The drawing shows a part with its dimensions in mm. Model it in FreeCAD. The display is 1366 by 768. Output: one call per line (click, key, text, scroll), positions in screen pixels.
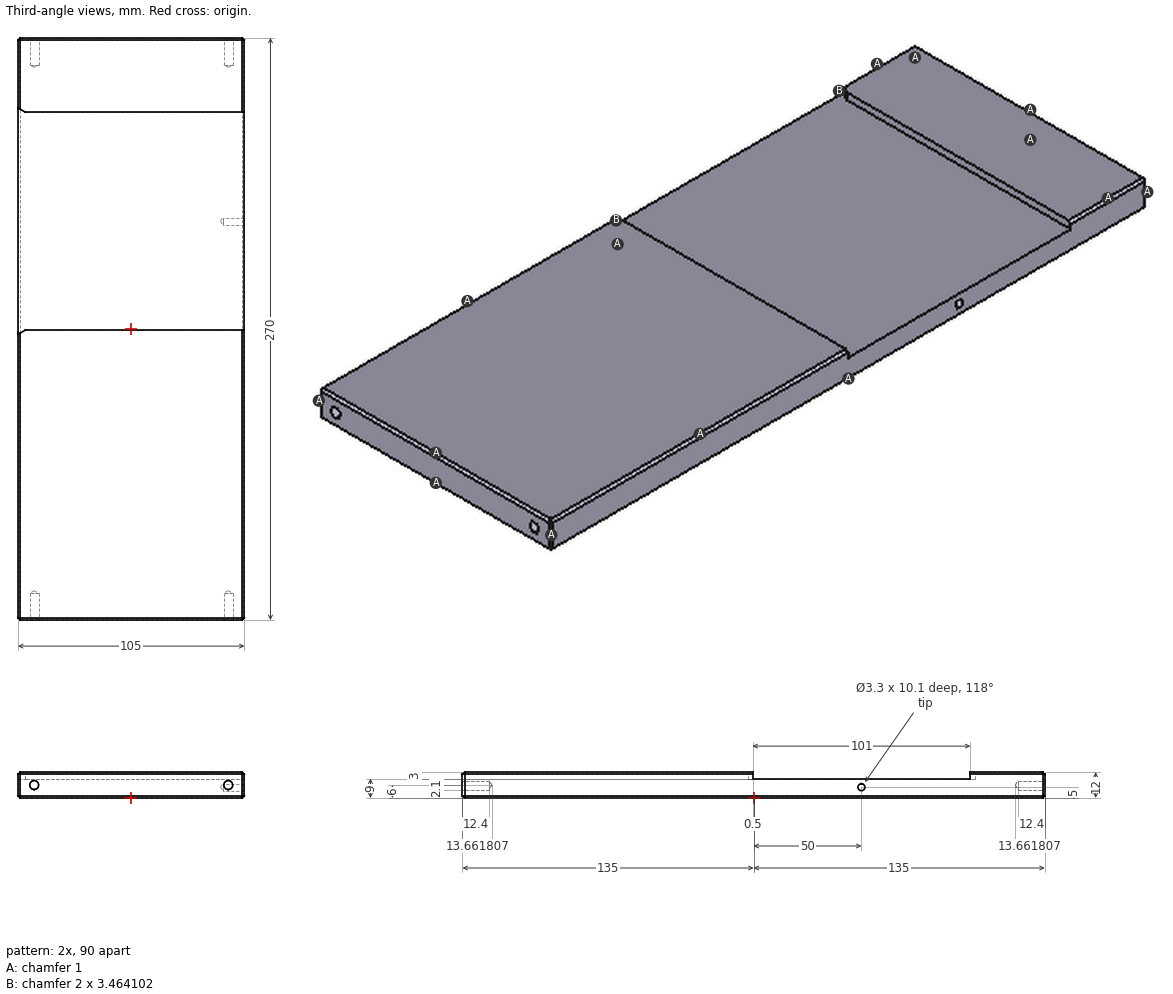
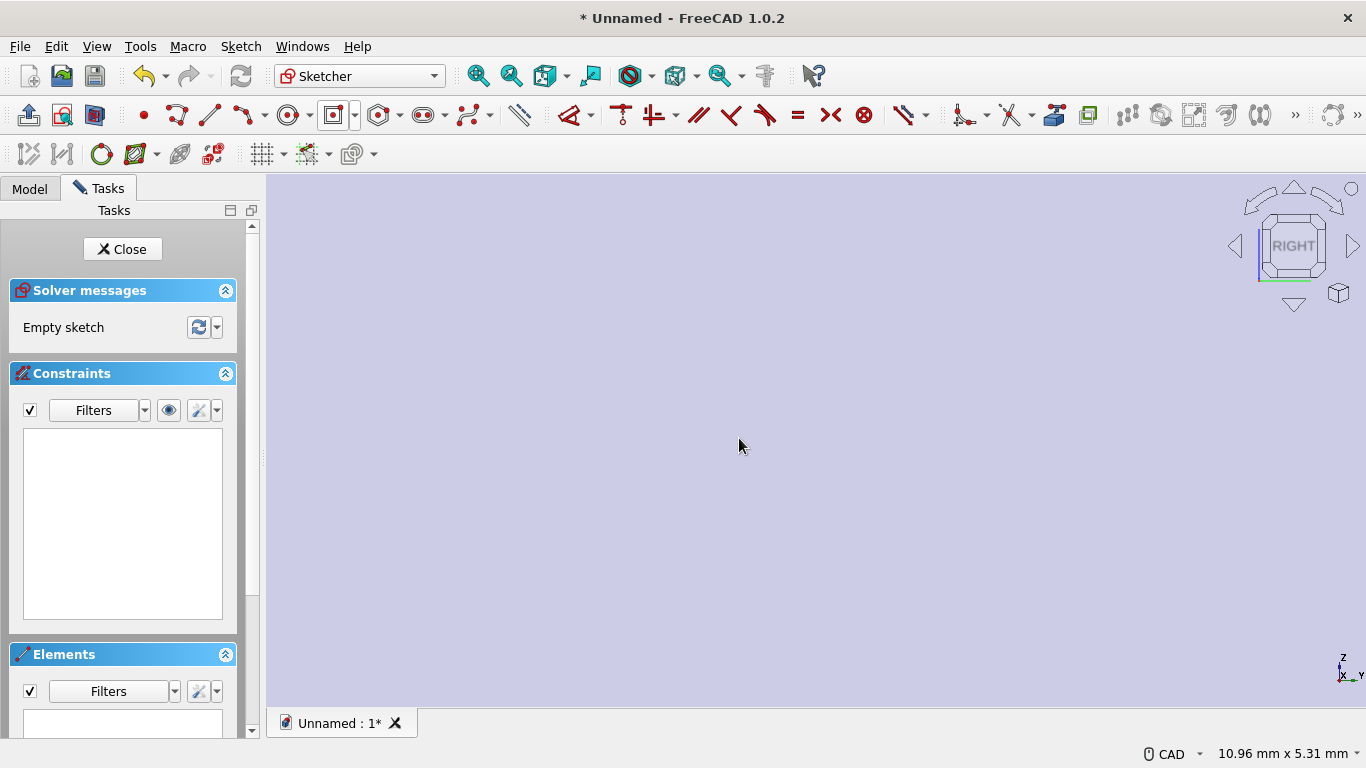
click(288, 116)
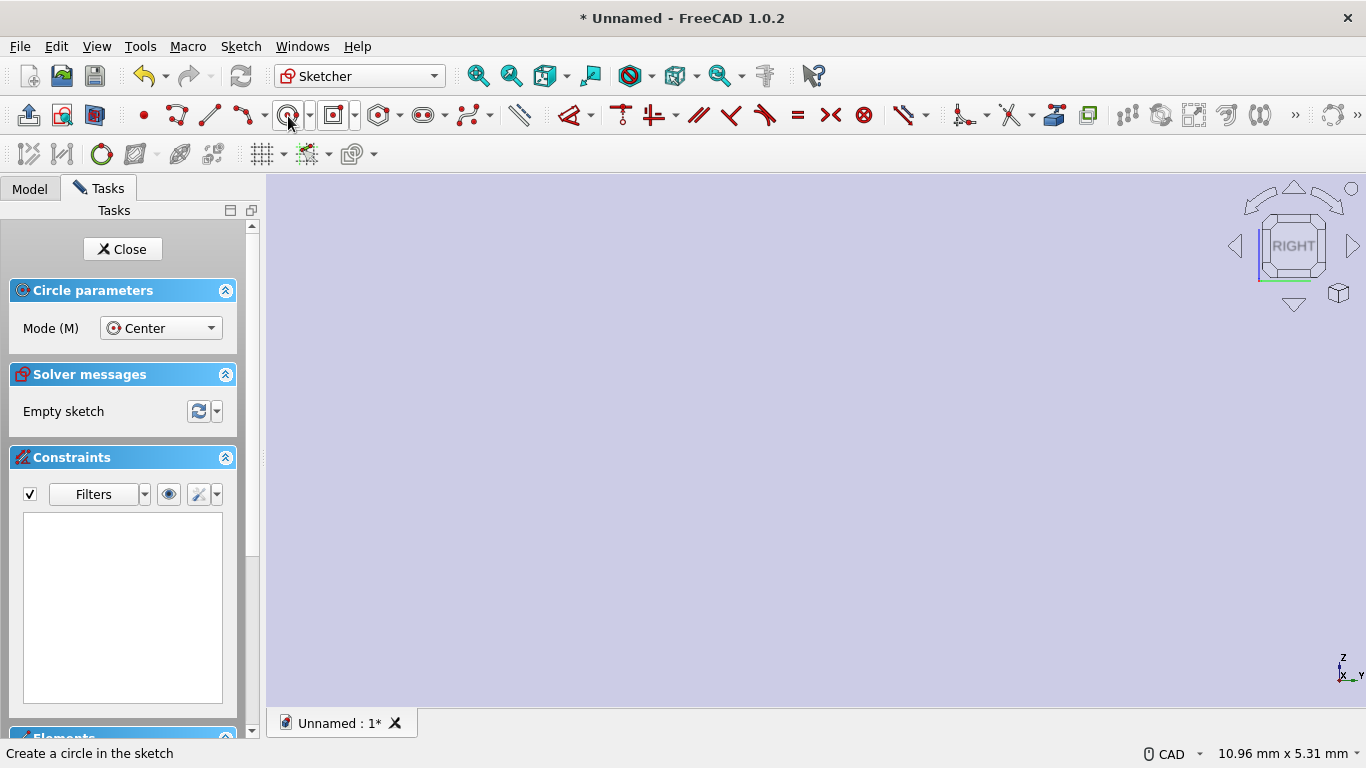
click(747, 440)
move(864, 323)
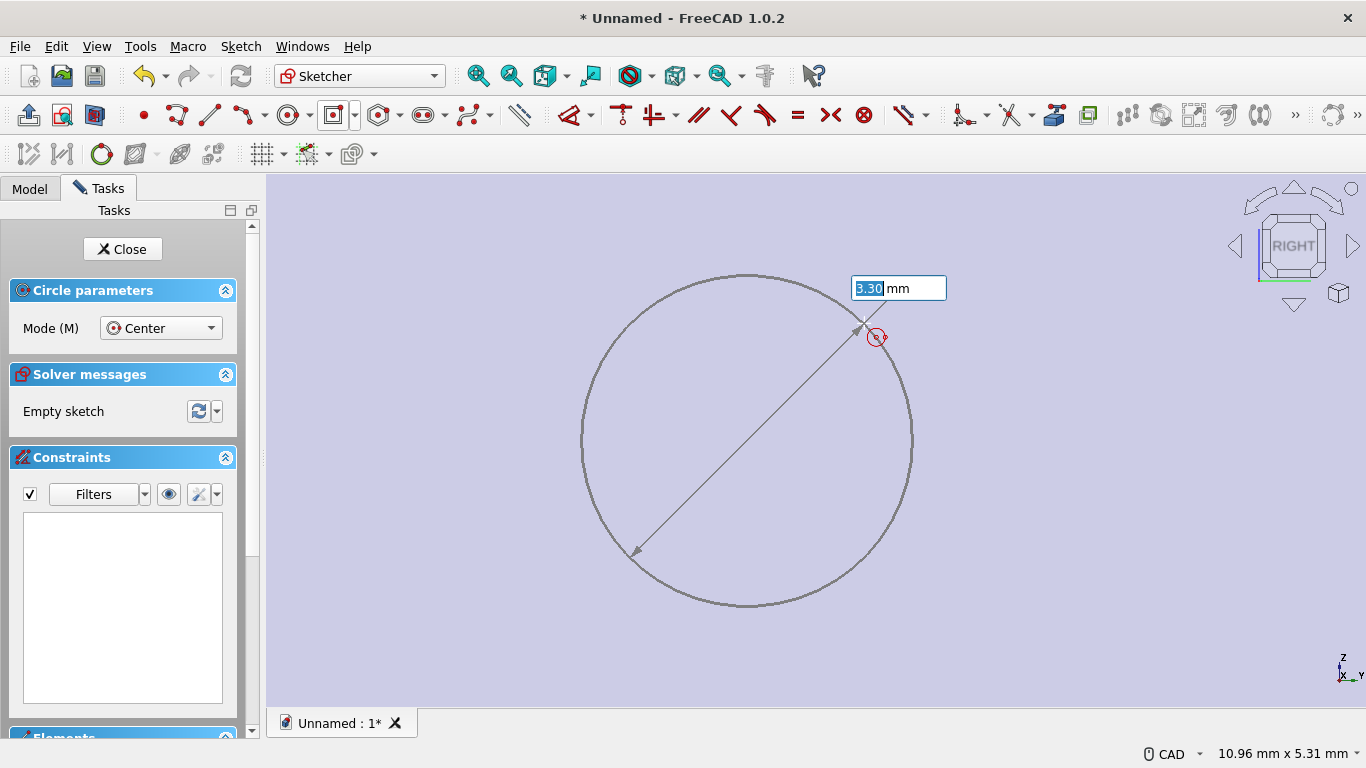
text(3.3)
key(Return)
key(Escape)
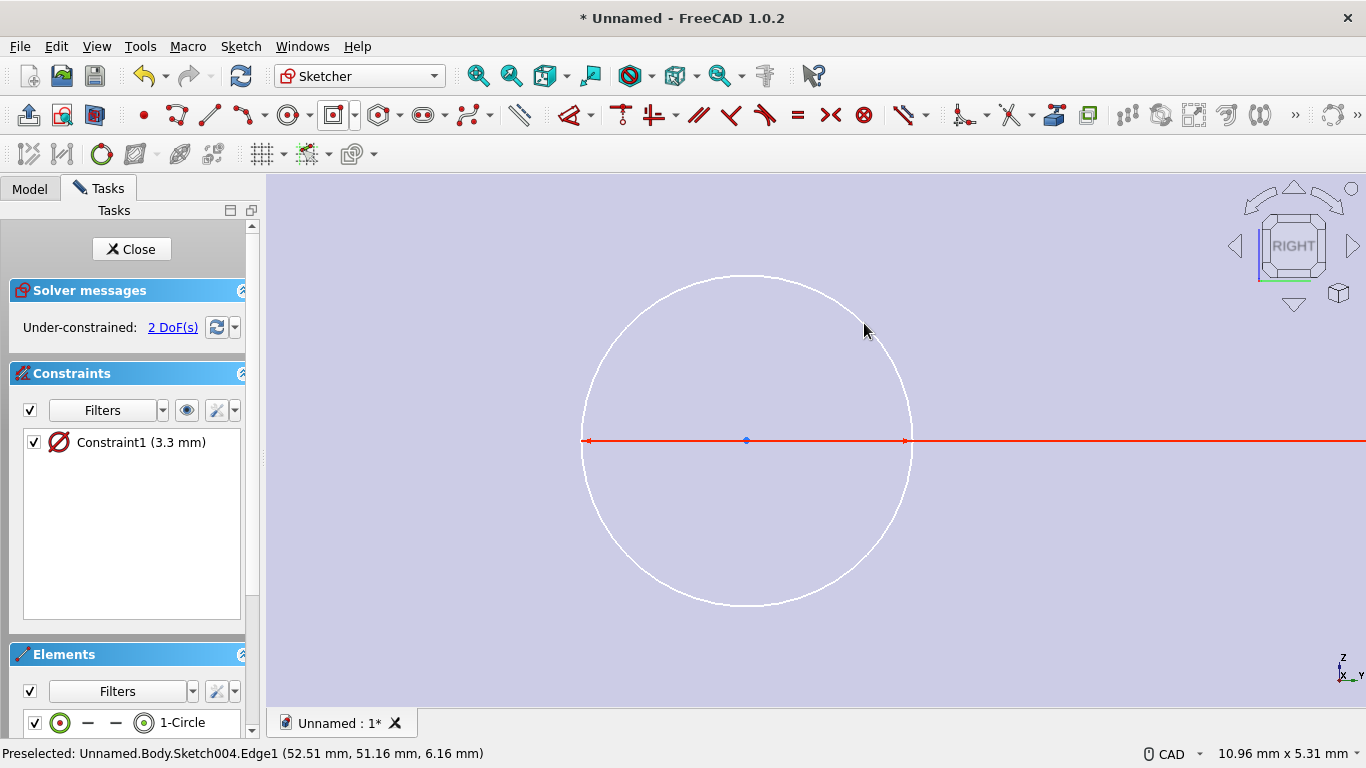
click(568, 116)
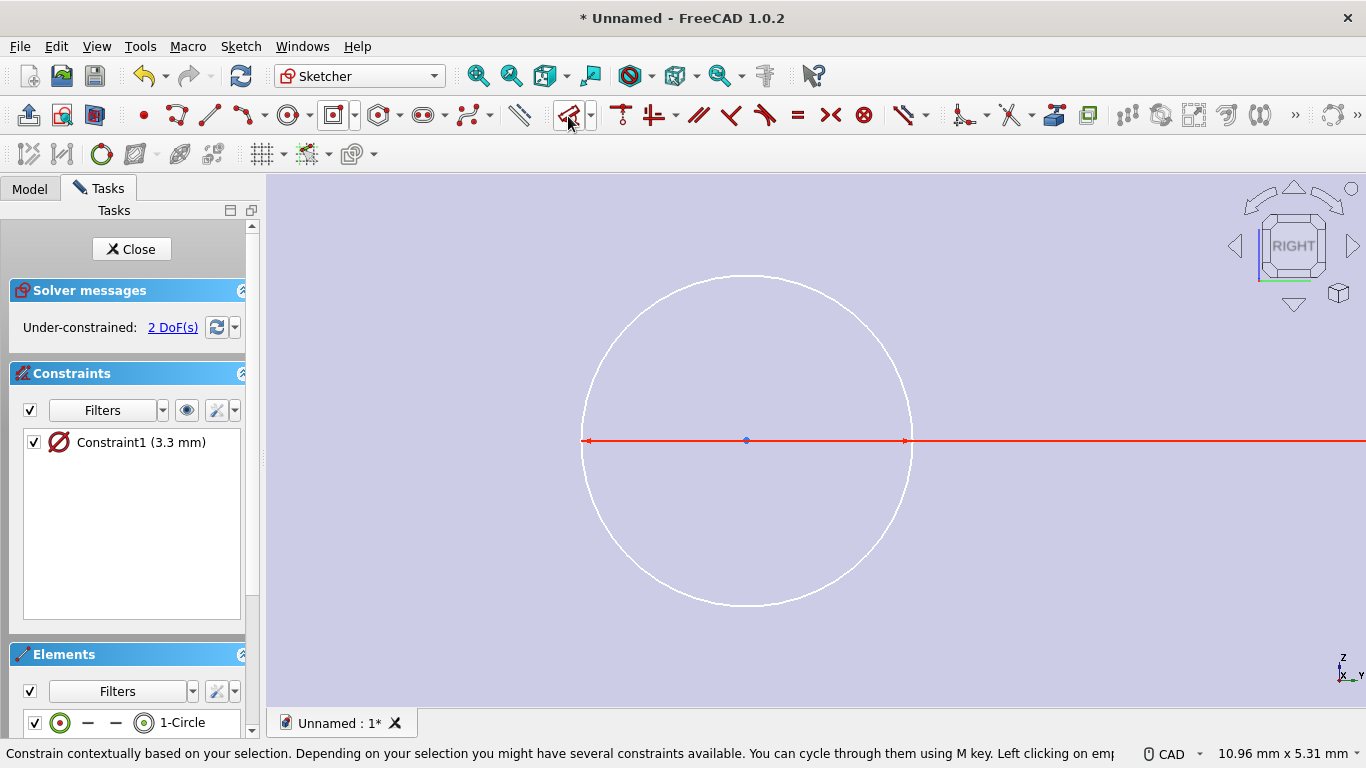
click(747, 441)
click(781, 560)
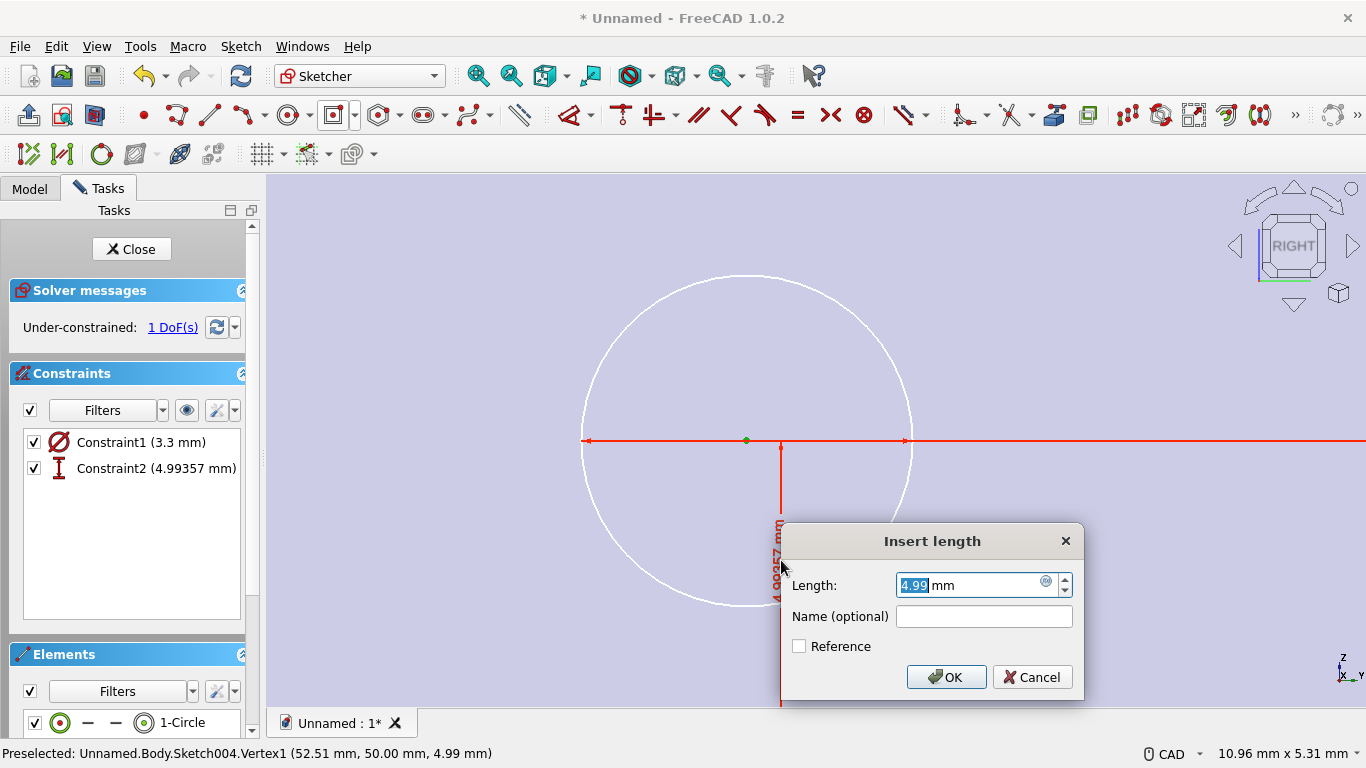
text(5)
key(Return)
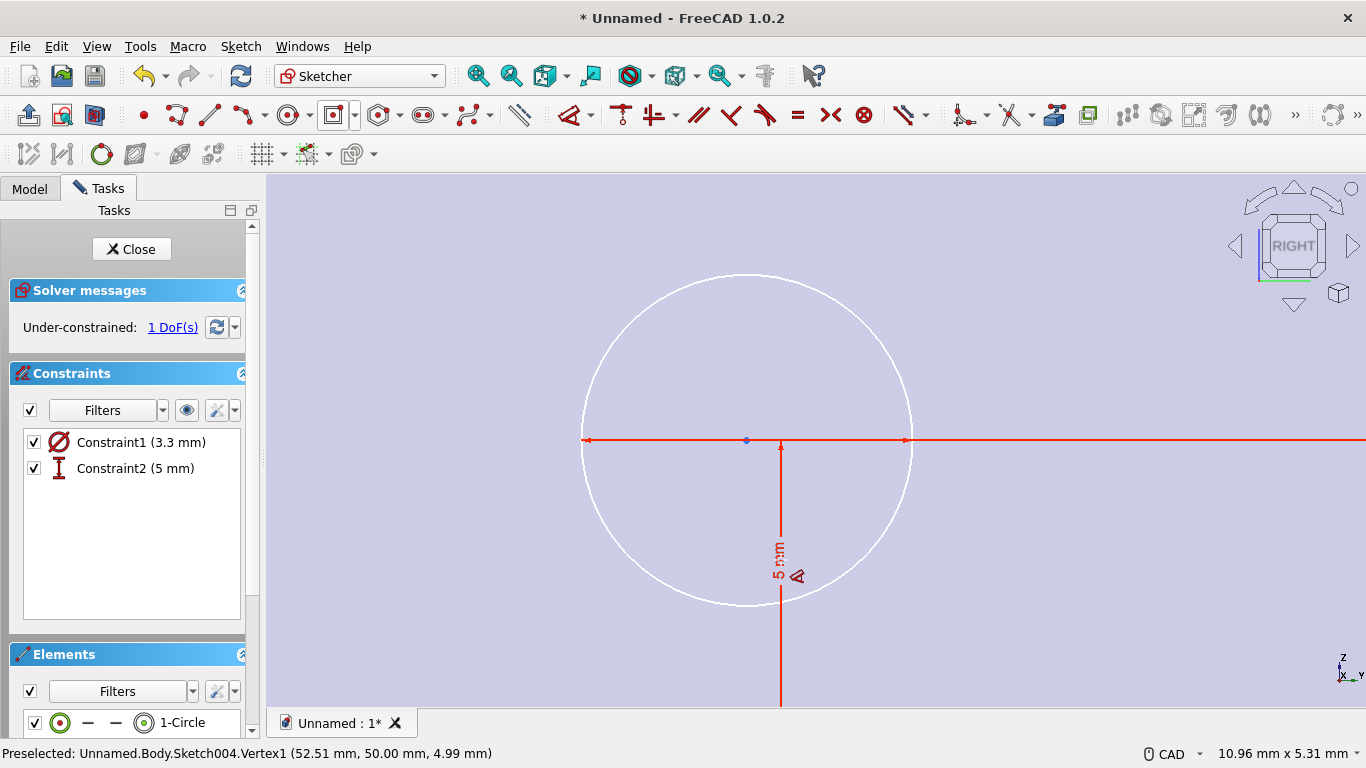
click(747, 440)
click(520, 406)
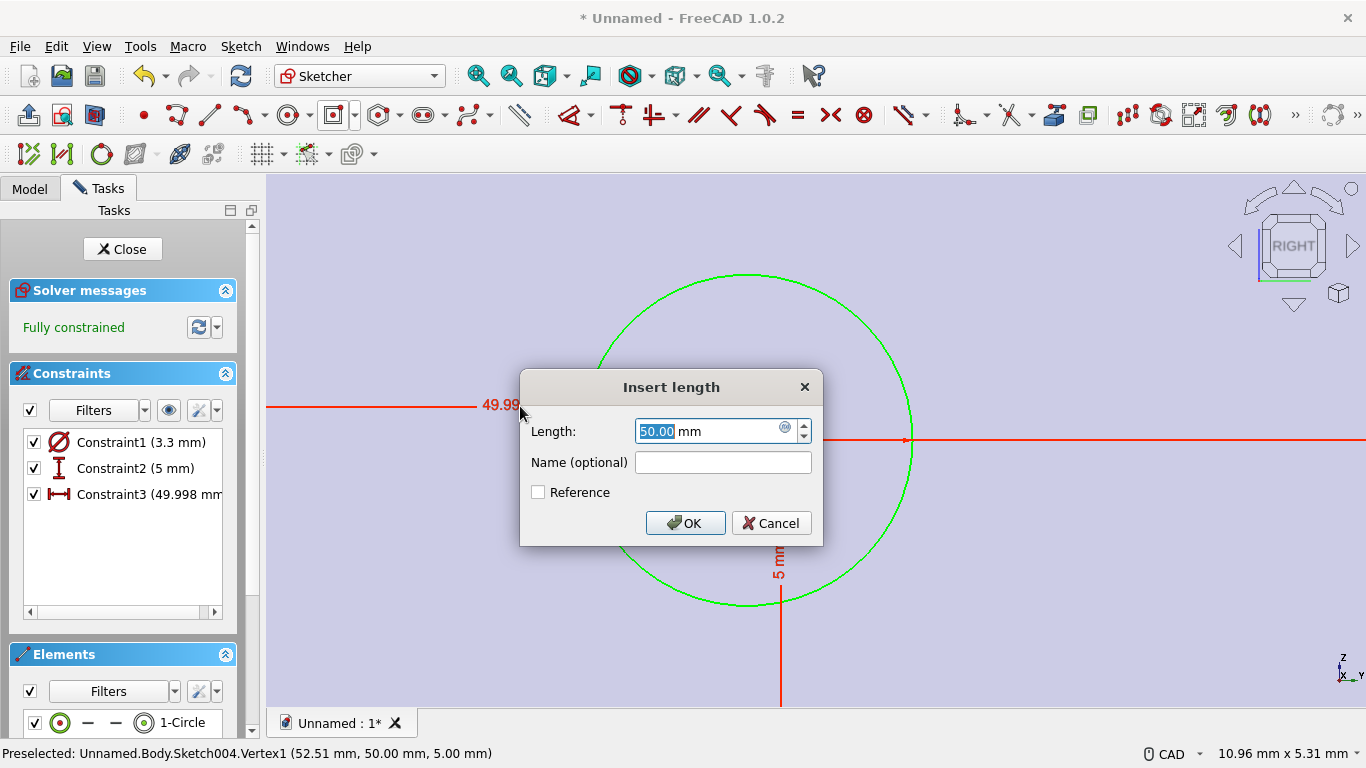
text(50)
key(Return)
key(Escape)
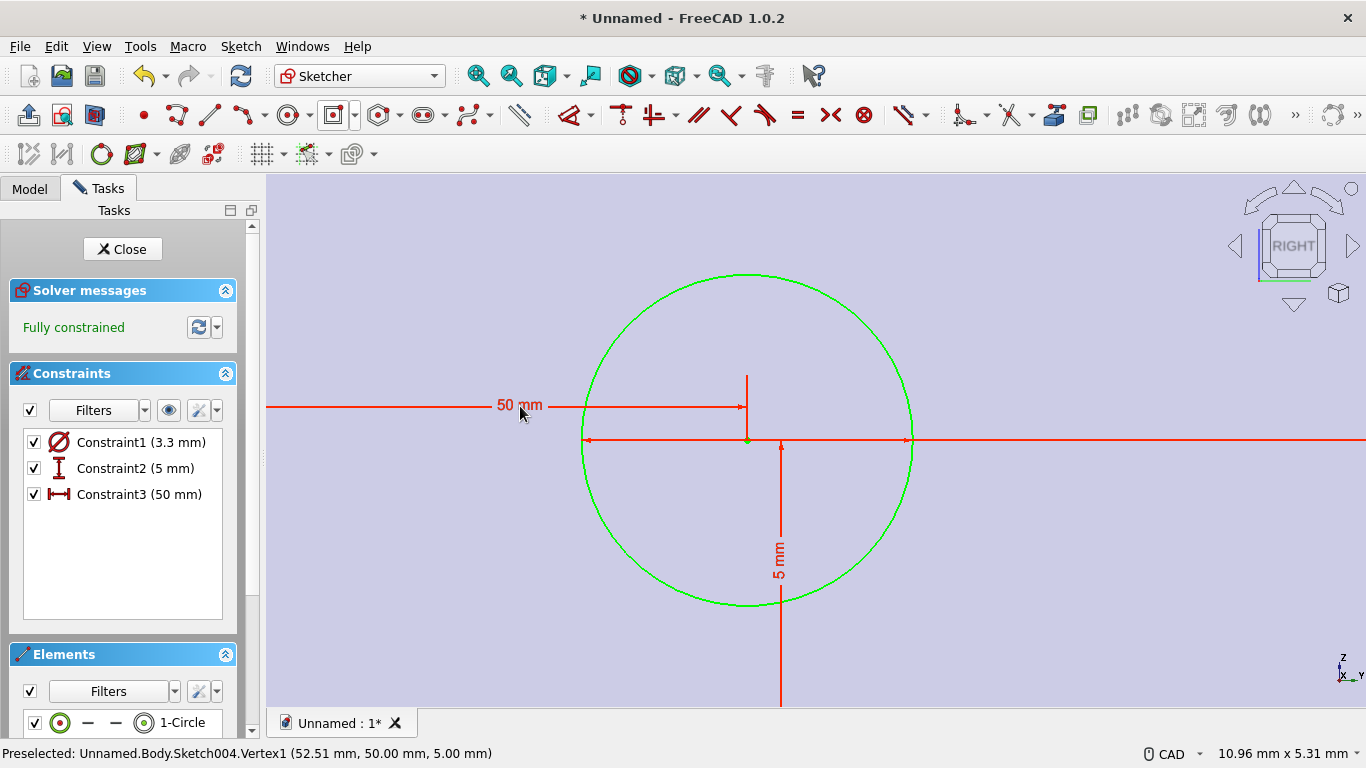
click(123, 249)